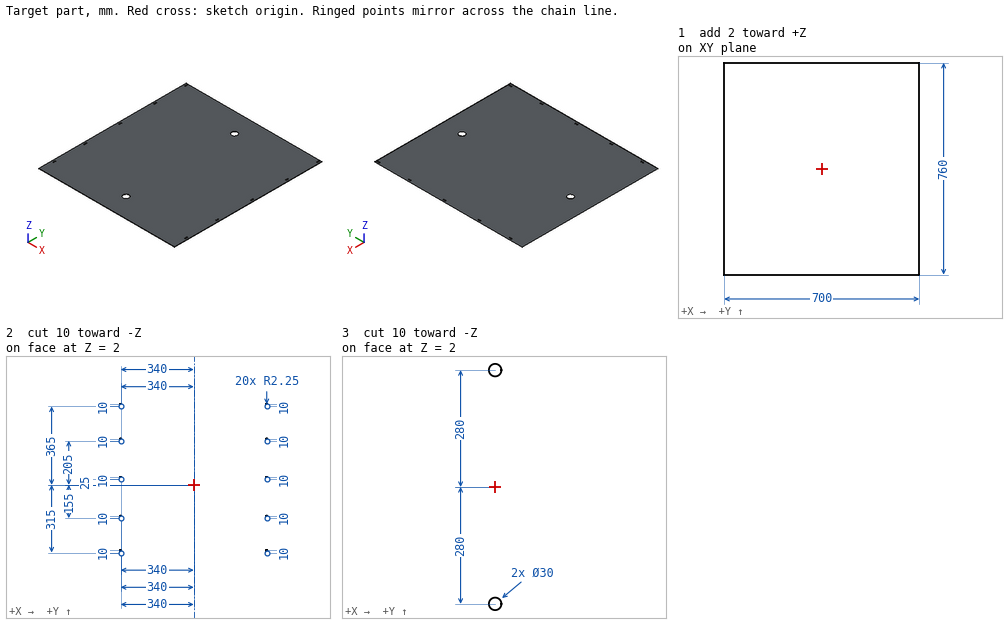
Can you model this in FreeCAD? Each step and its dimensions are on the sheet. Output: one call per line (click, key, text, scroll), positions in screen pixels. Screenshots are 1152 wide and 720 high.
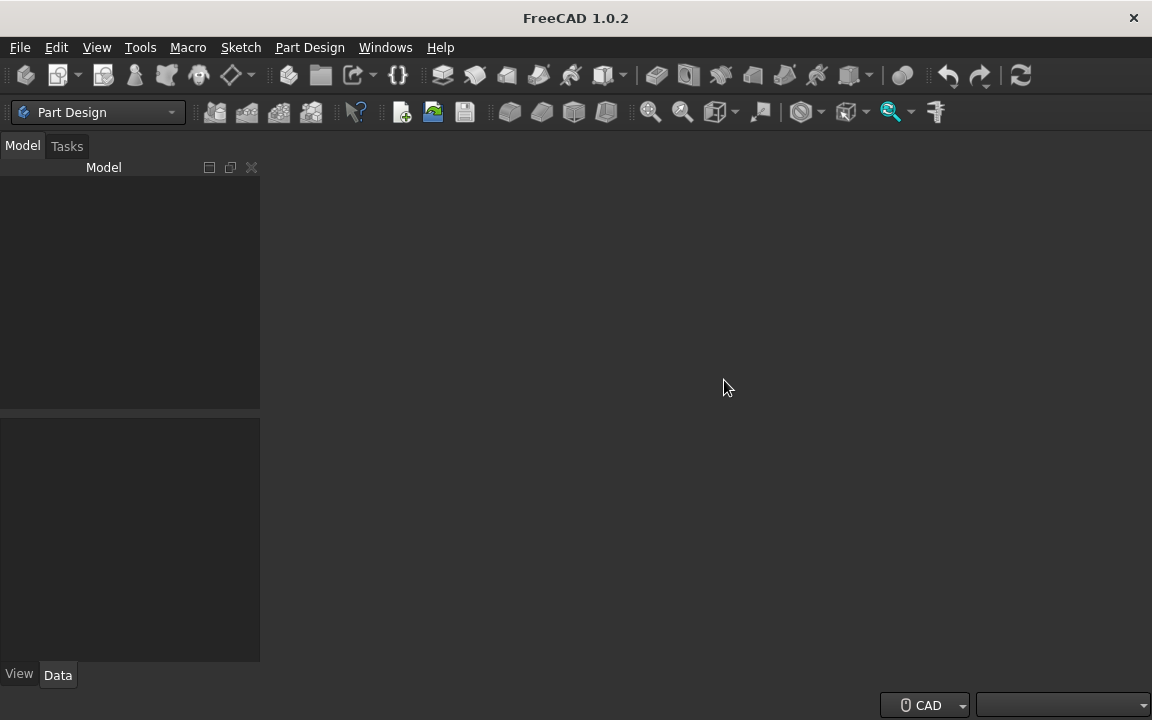
key(ctrl+n)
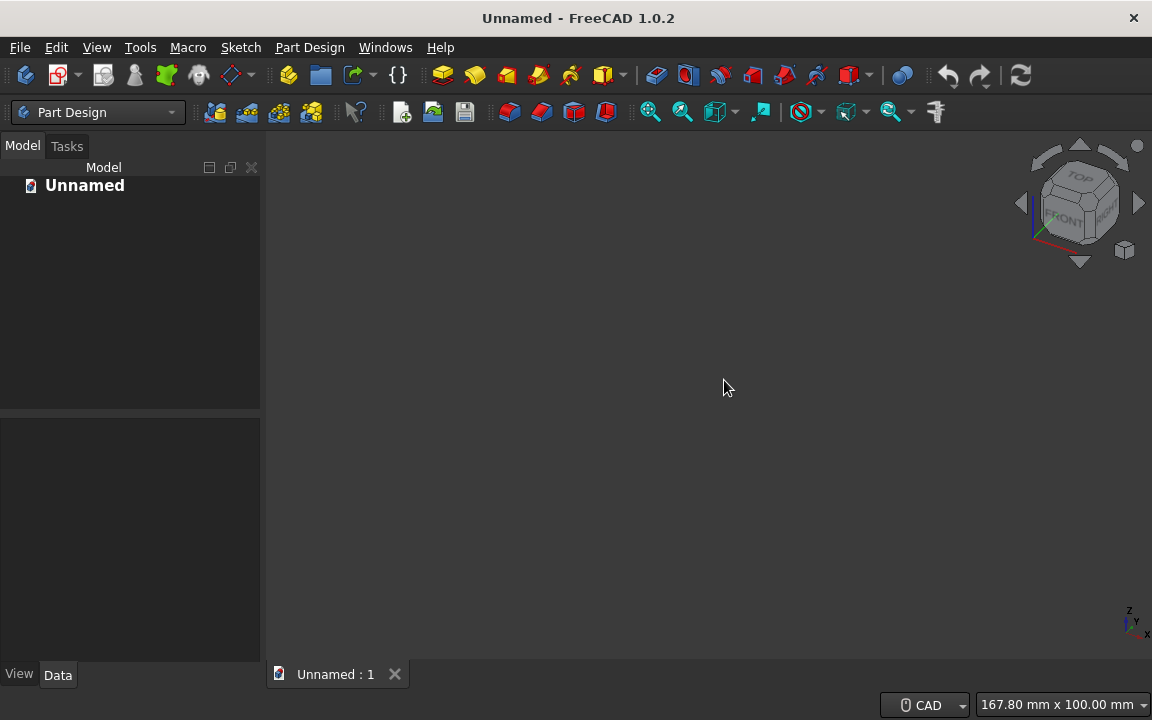
click(58, 76)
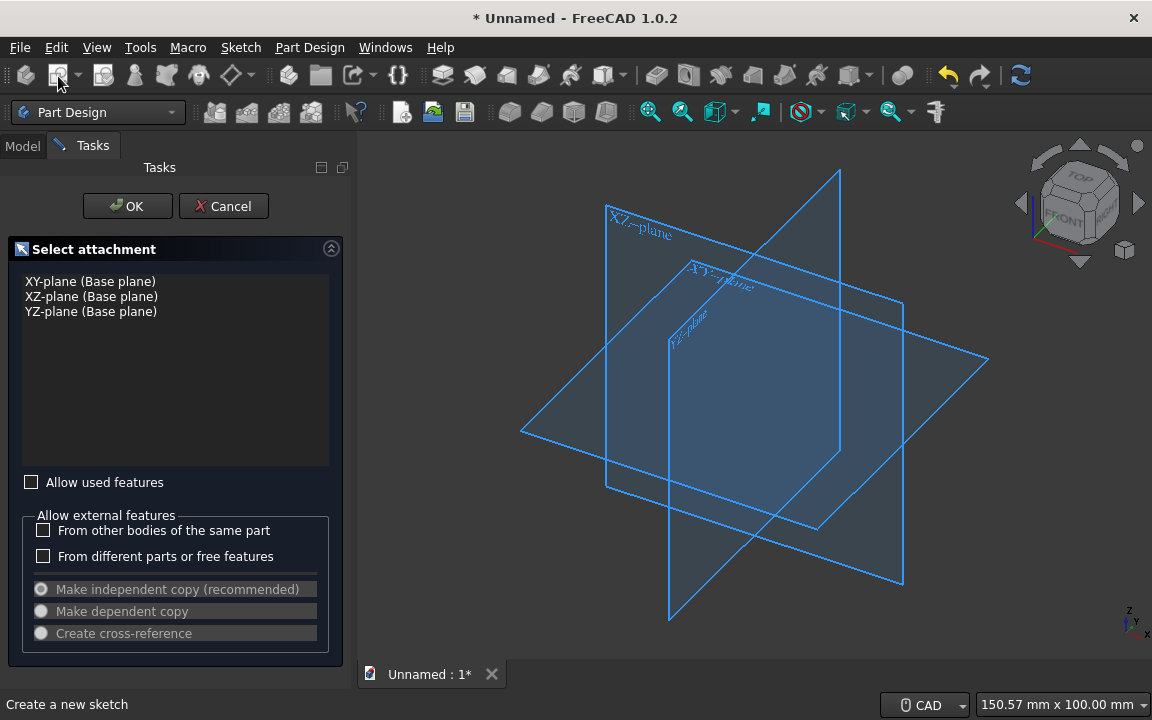
click(82, 282)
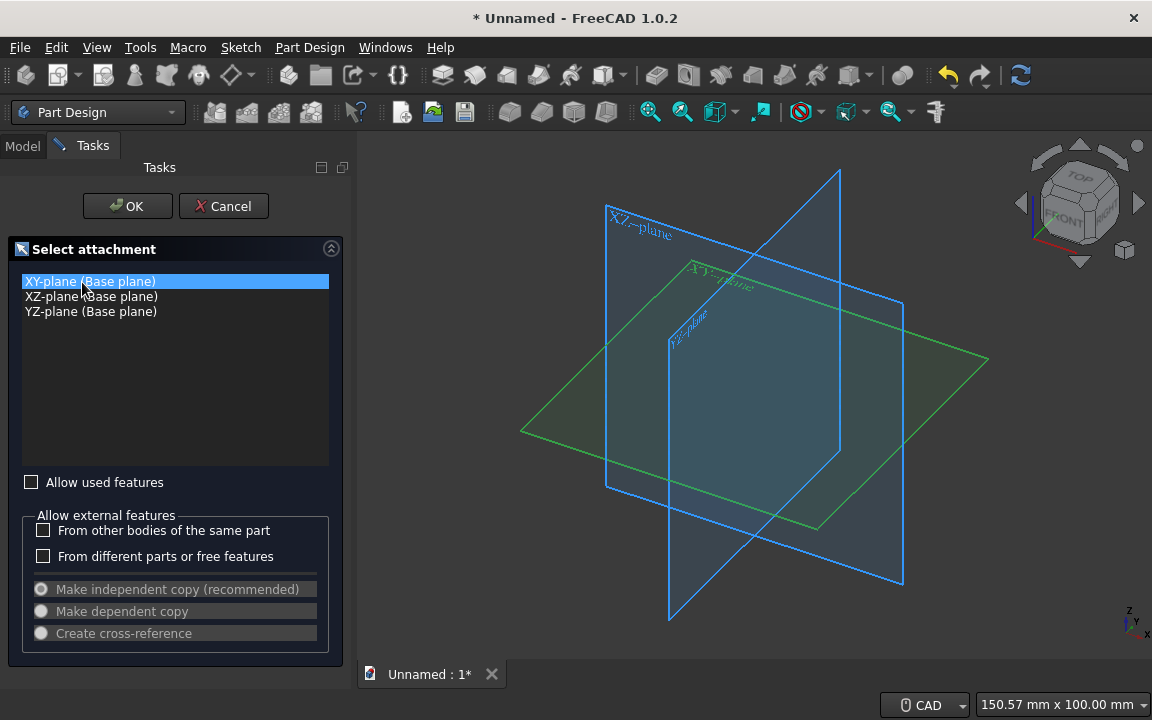
click(128, 206)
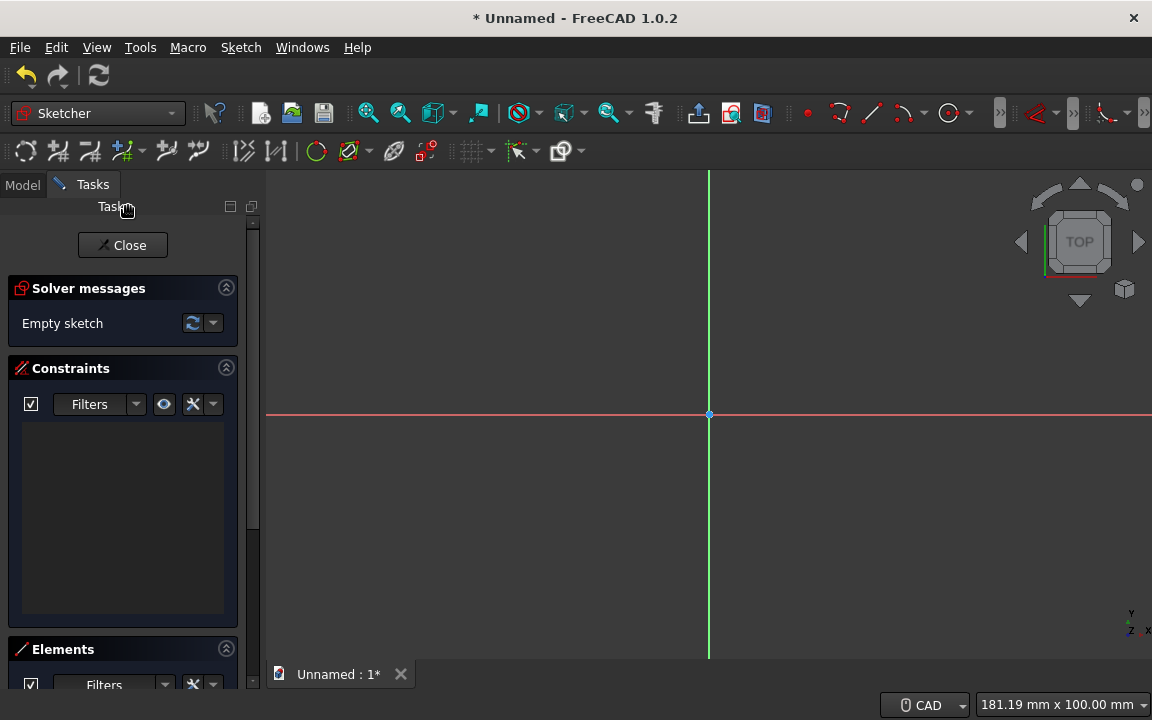
scroll(634, 414, down, 12)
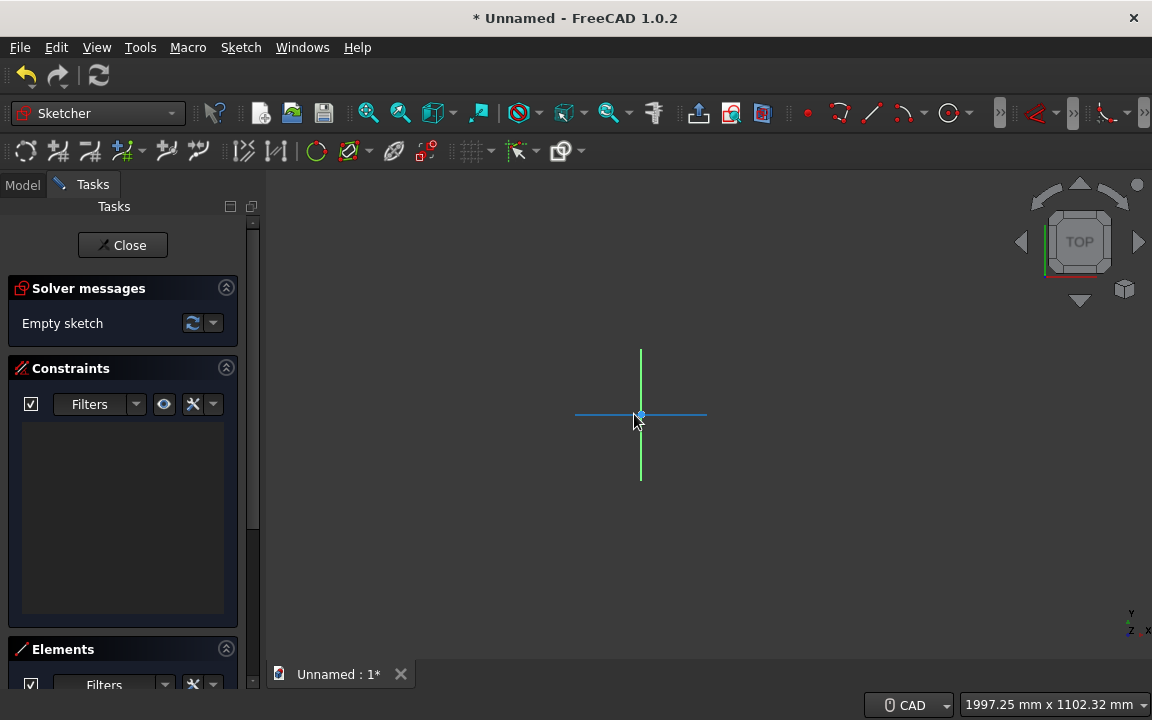
key(g)
key(v)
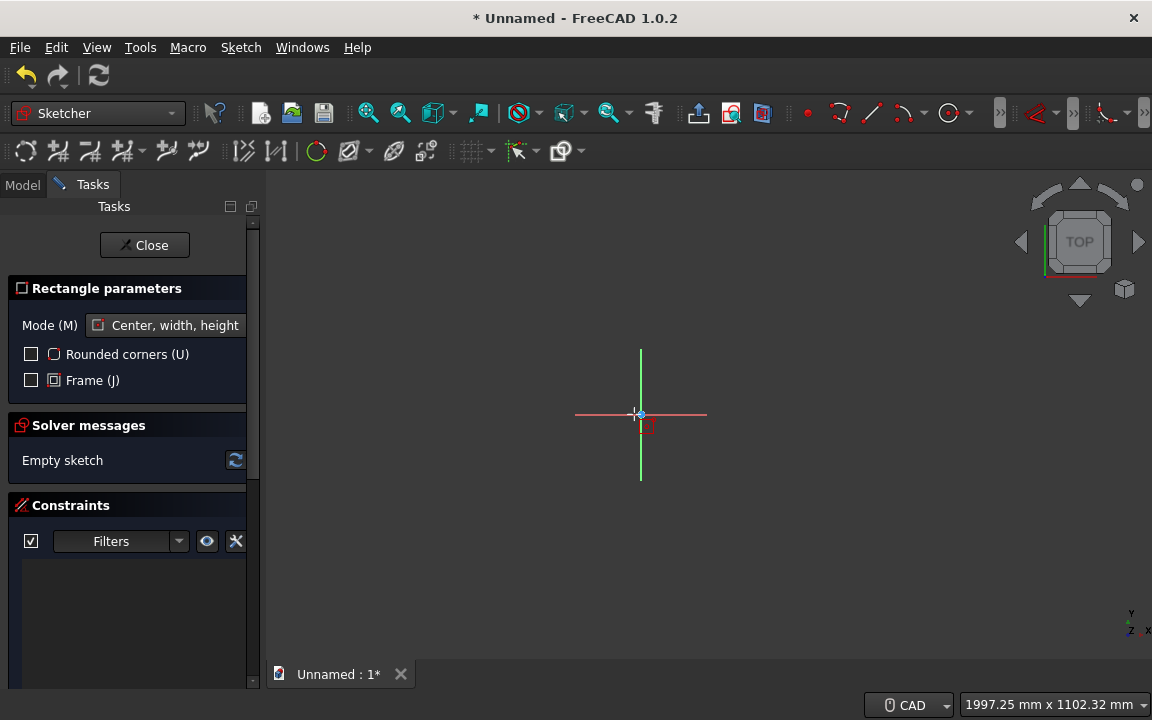
click(641, 414)
move(796, 246)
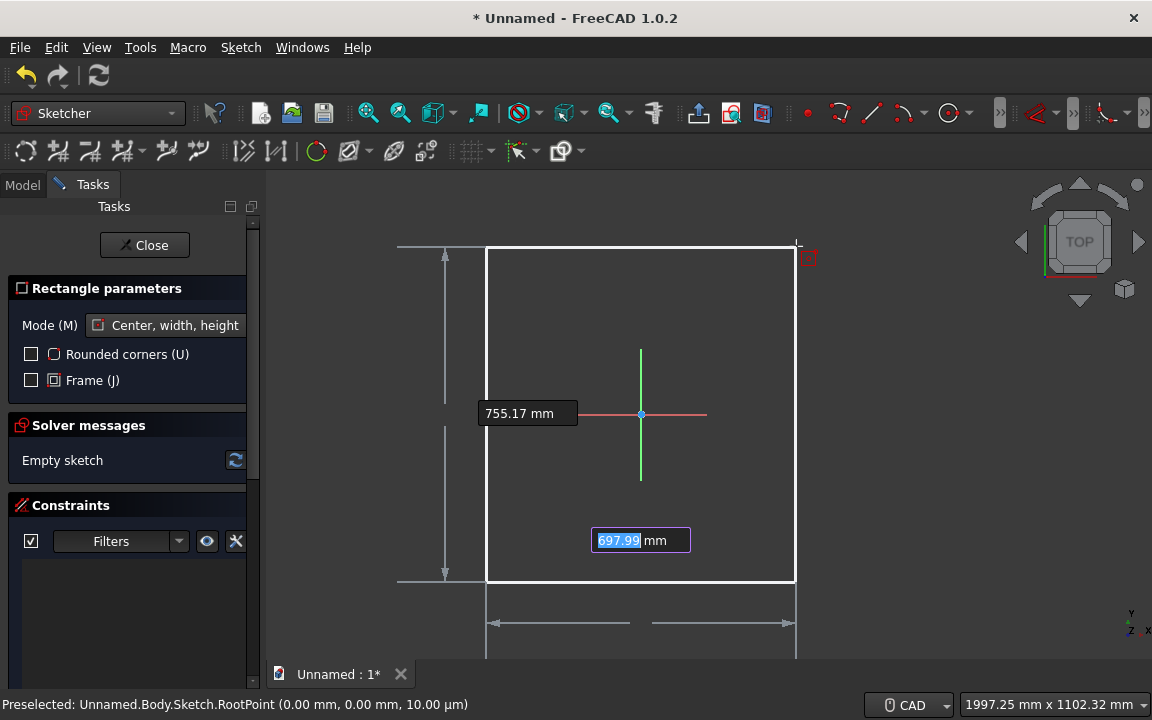
text(700)
key(Tab)
text(760)
key(Return)
key(Escape)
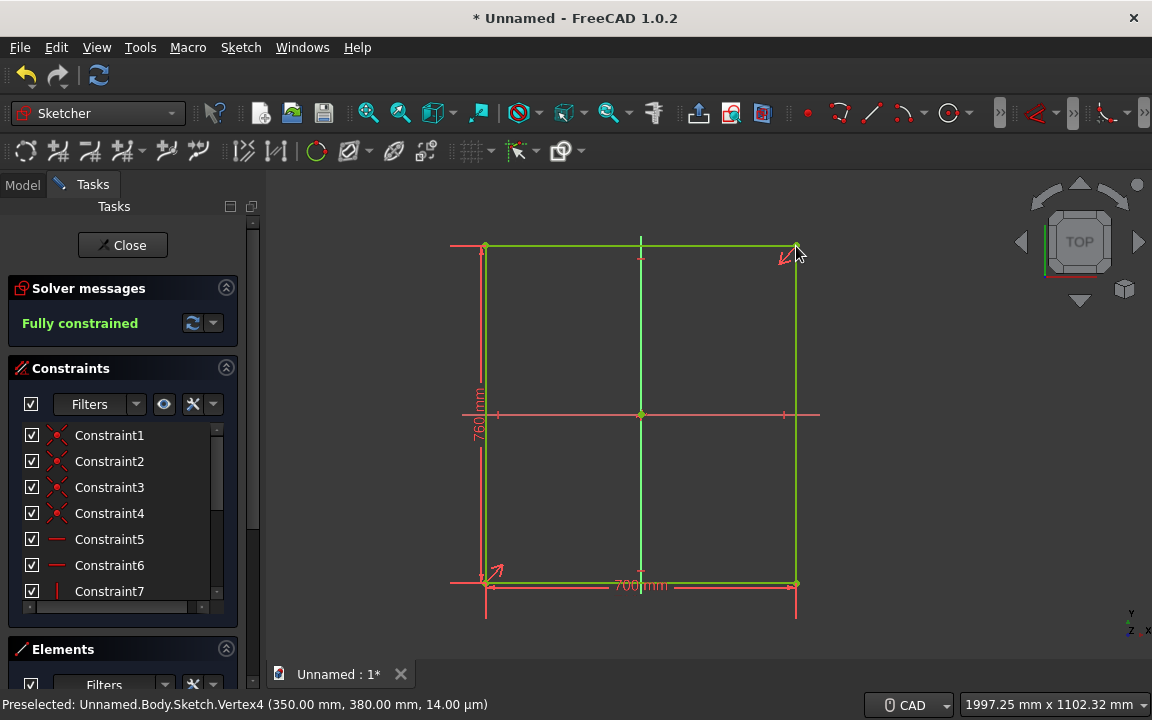
click(123, 245)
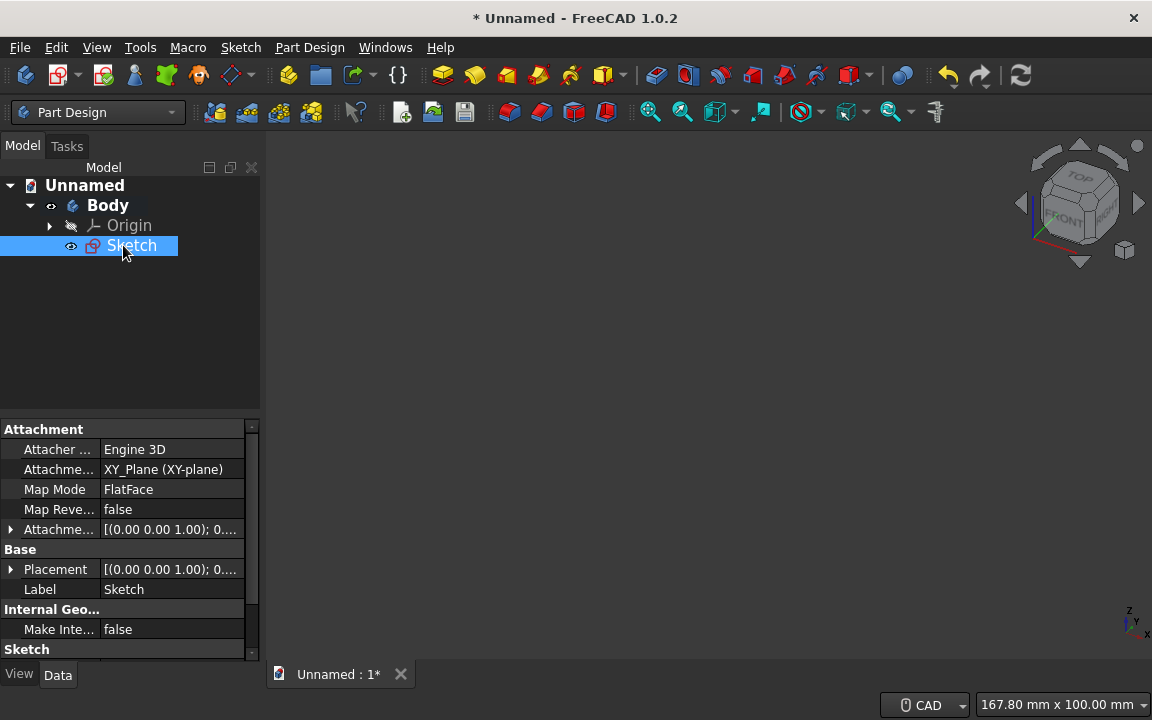
click(444, 76)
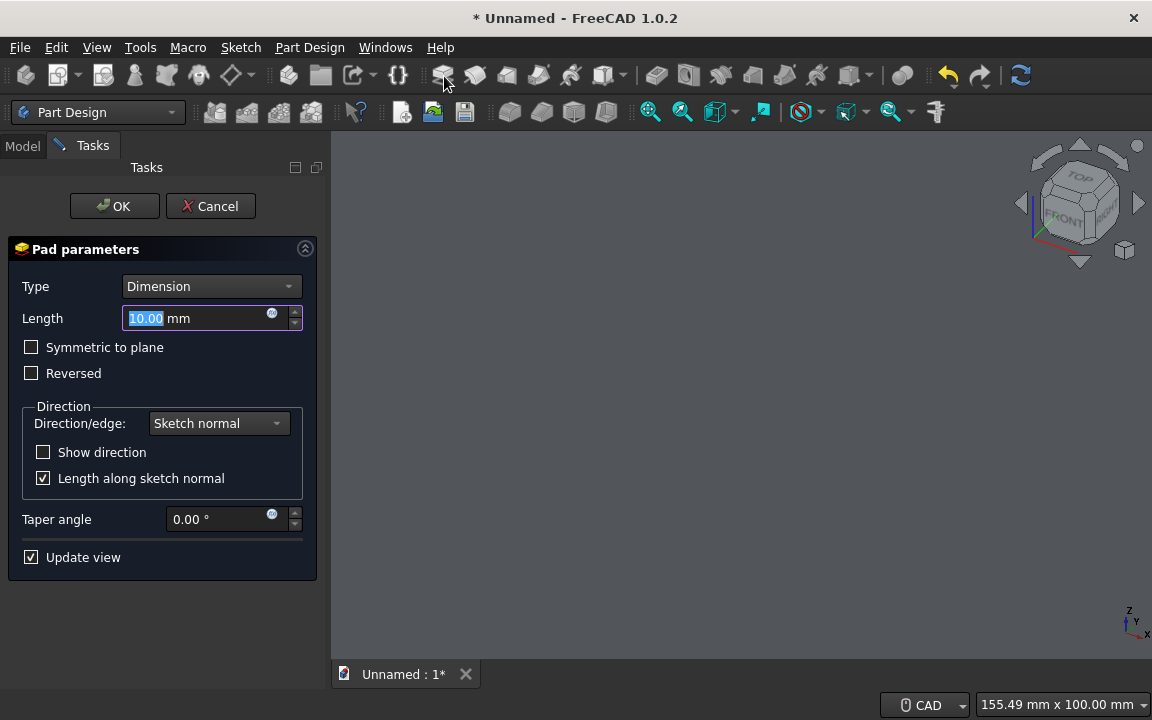
text(2)
key(Tab)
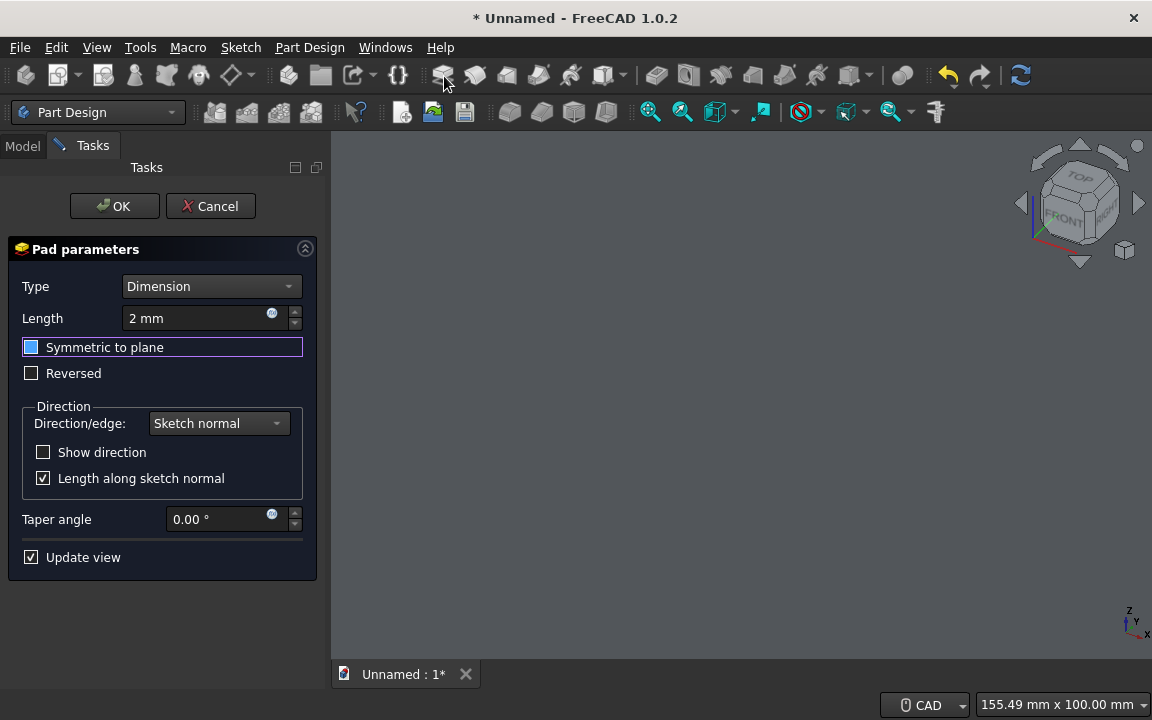
click(115, 206)